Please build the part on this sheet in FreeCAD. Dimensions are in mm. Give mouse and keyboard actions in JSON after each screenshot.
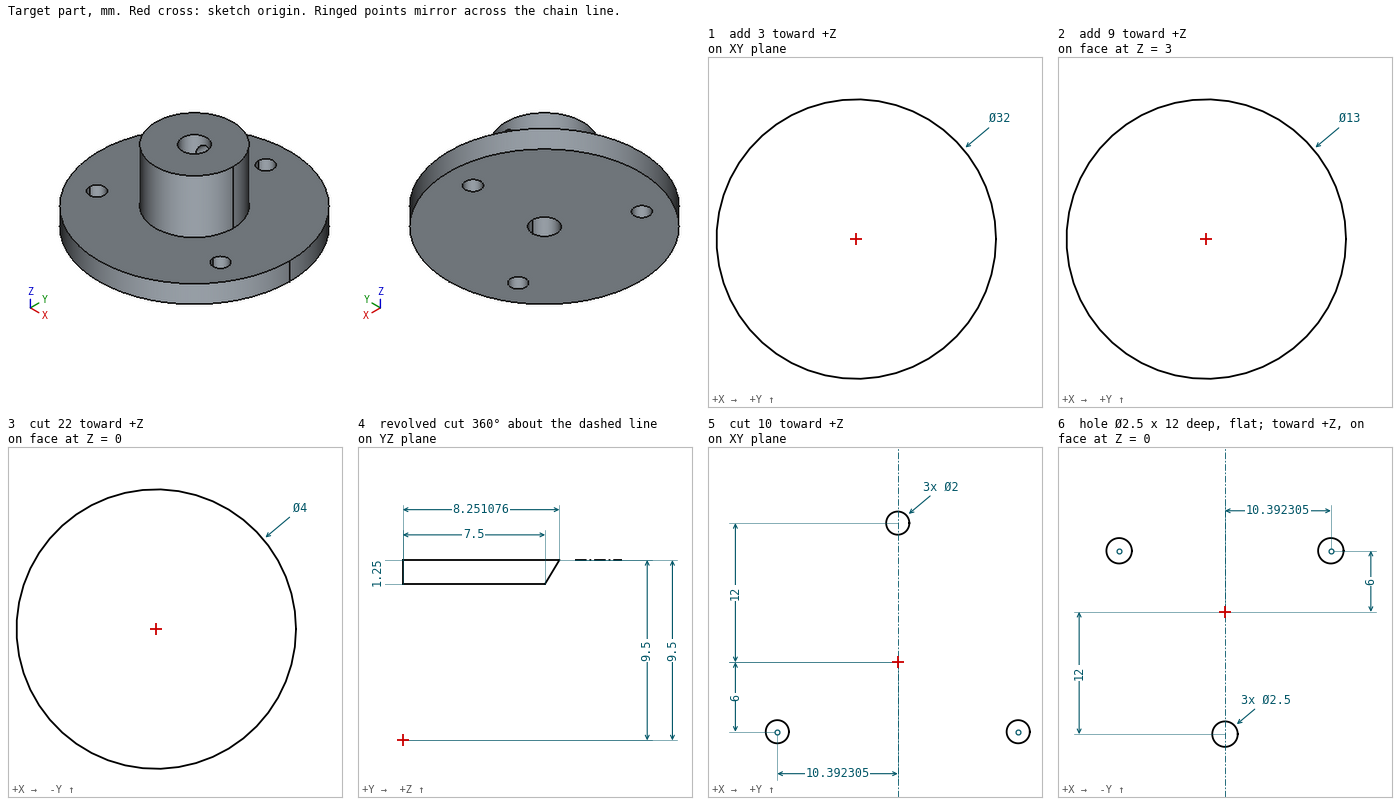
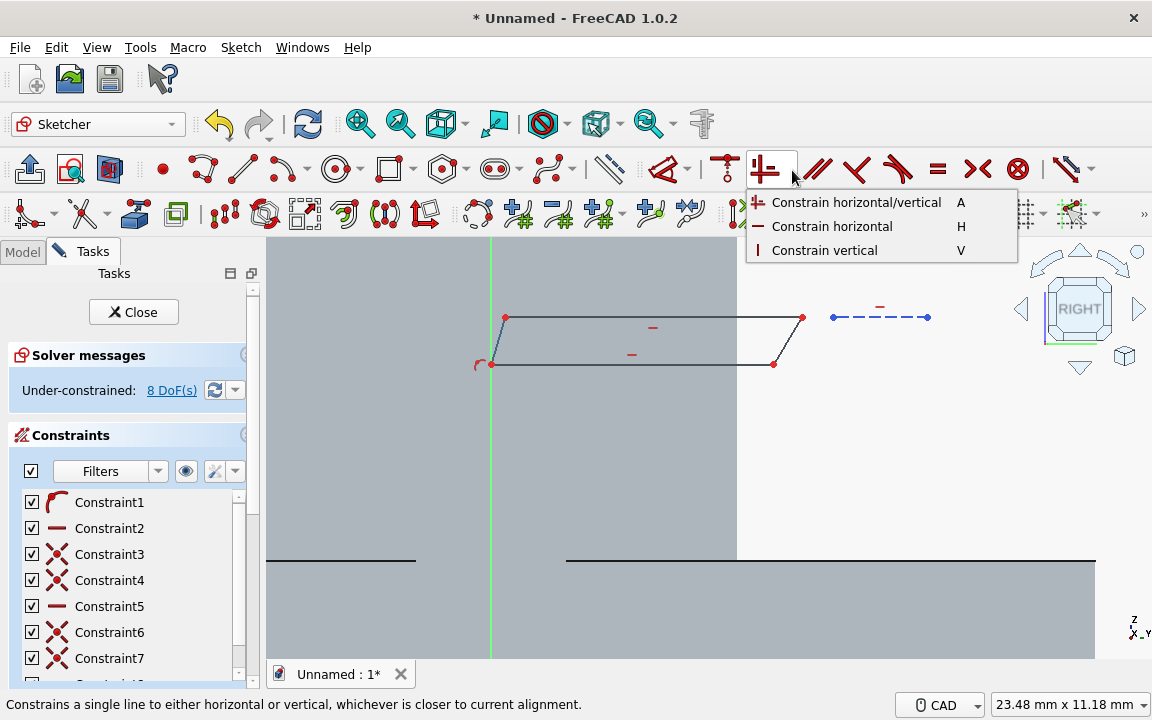
{"action": "left_click", "coordinate": [882, 250]}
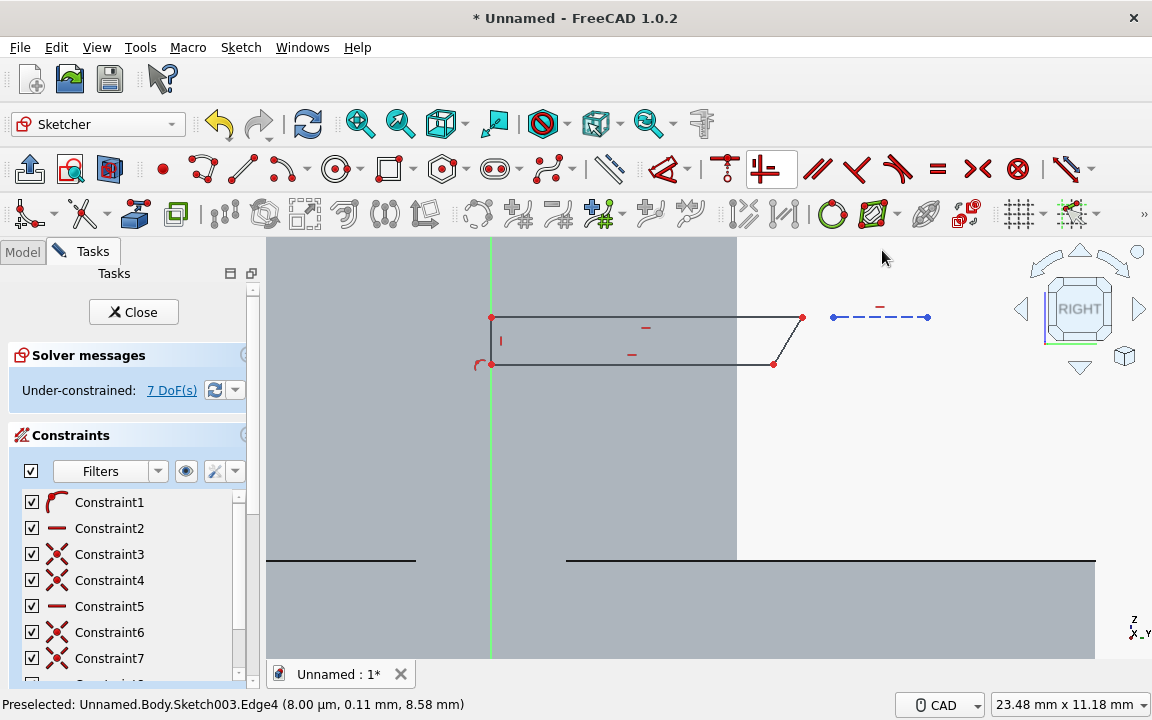
{"action": "left_click", "coordinate": [664, 170]}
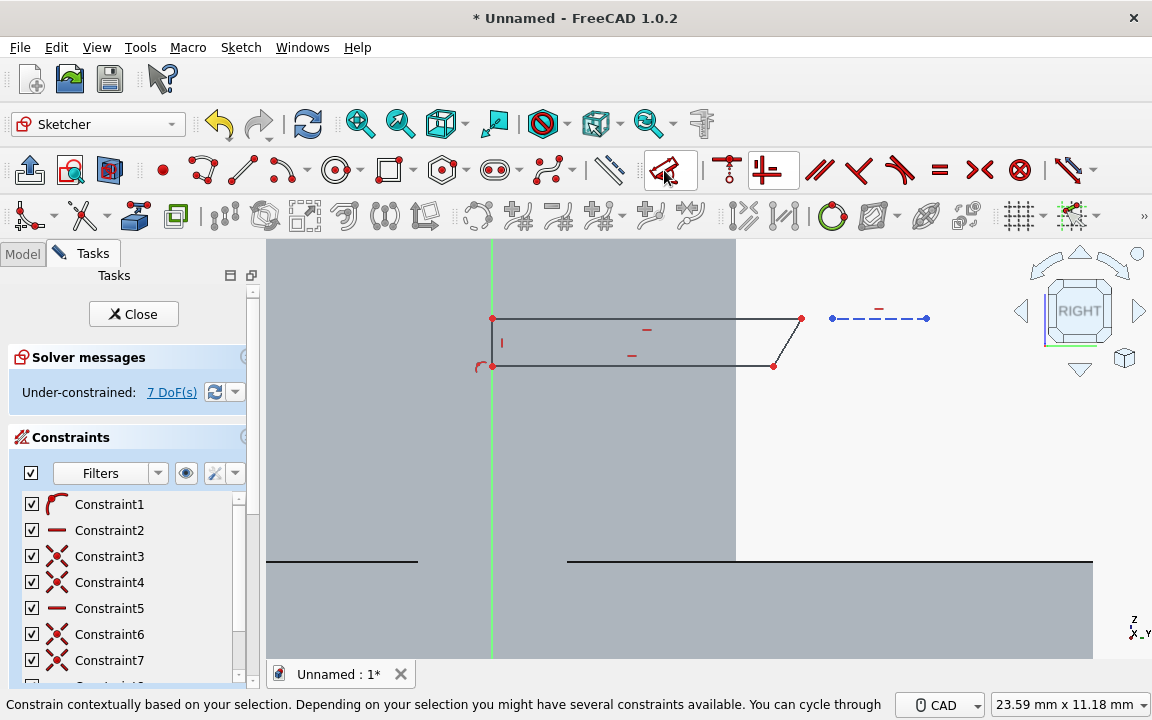
{"action": "left_click", "coordinate": [577, 366]}
{"action": "left_click", "coordinate": [633, 332]}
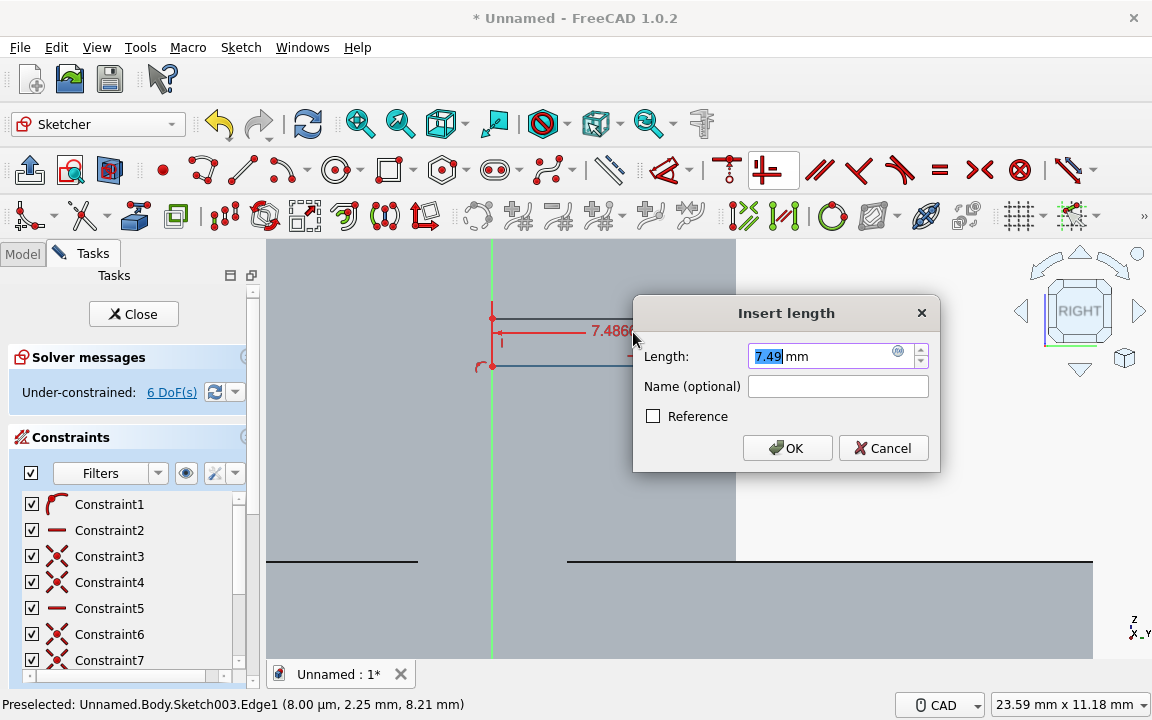
{"action": "type", "text": "7.5"}
{"action": "key", "text": "Return"}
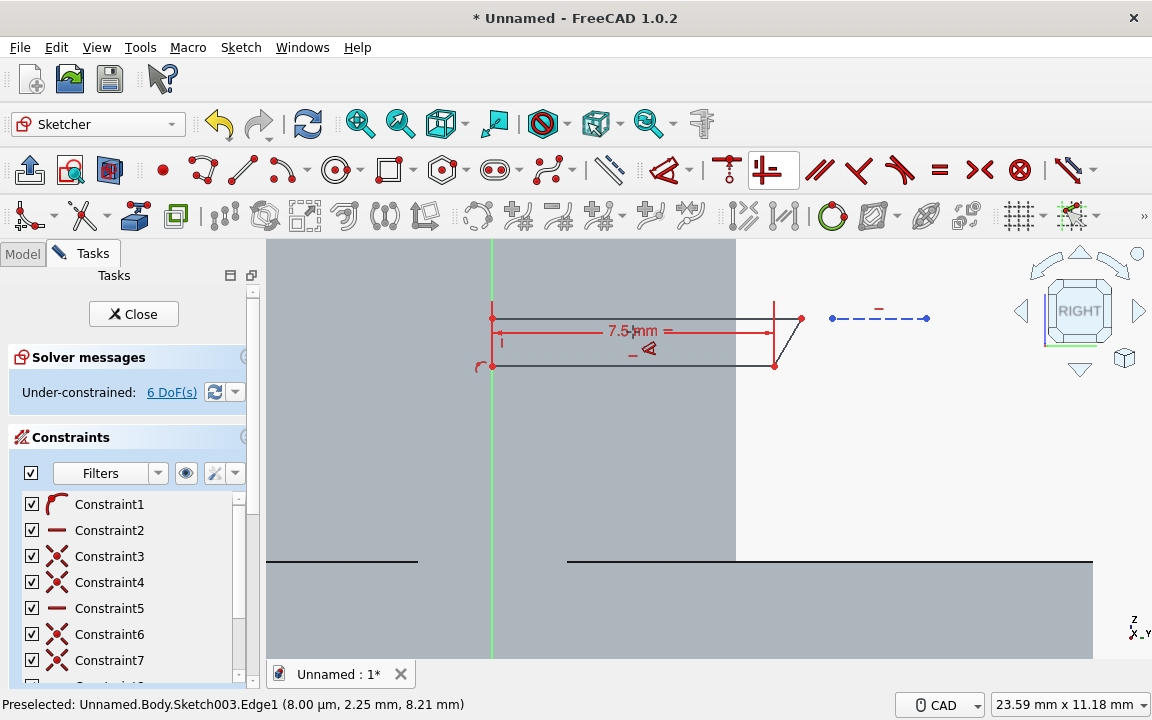
{"action": "left_click", "coordinate": [492, 333]}
{"action": "left_click", "coordinate": [458, 342]}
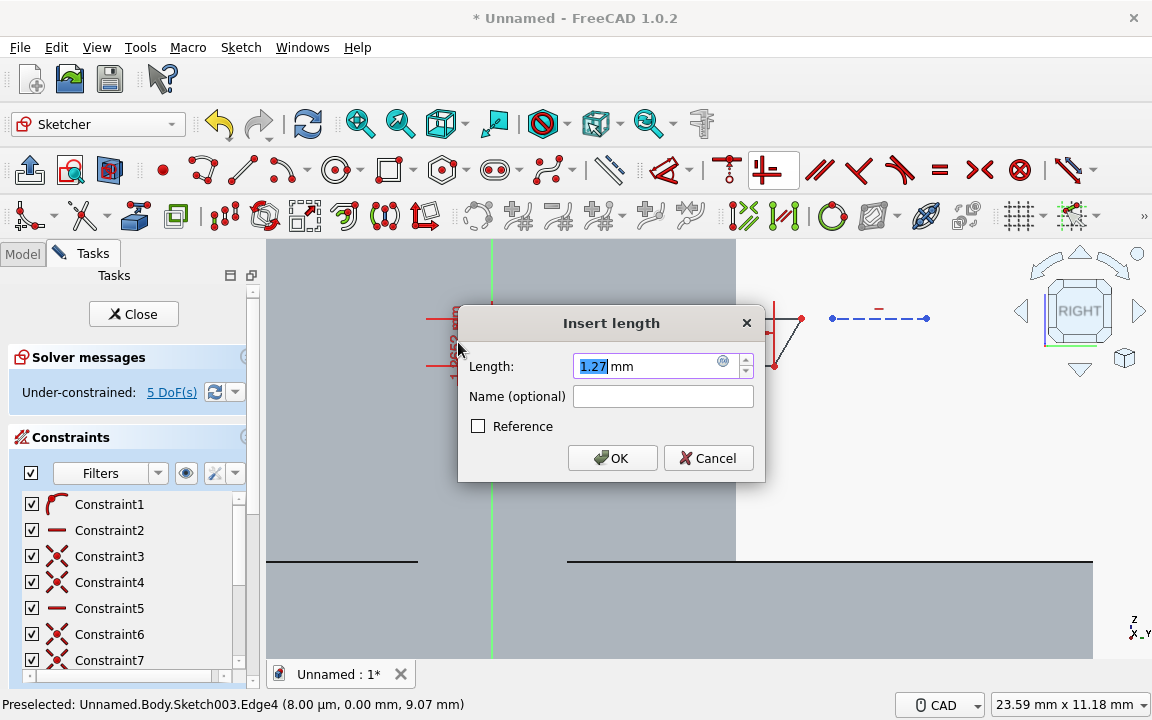
{"action": "type", "text": "1.25"}
{"action": "key", "text": "Return"}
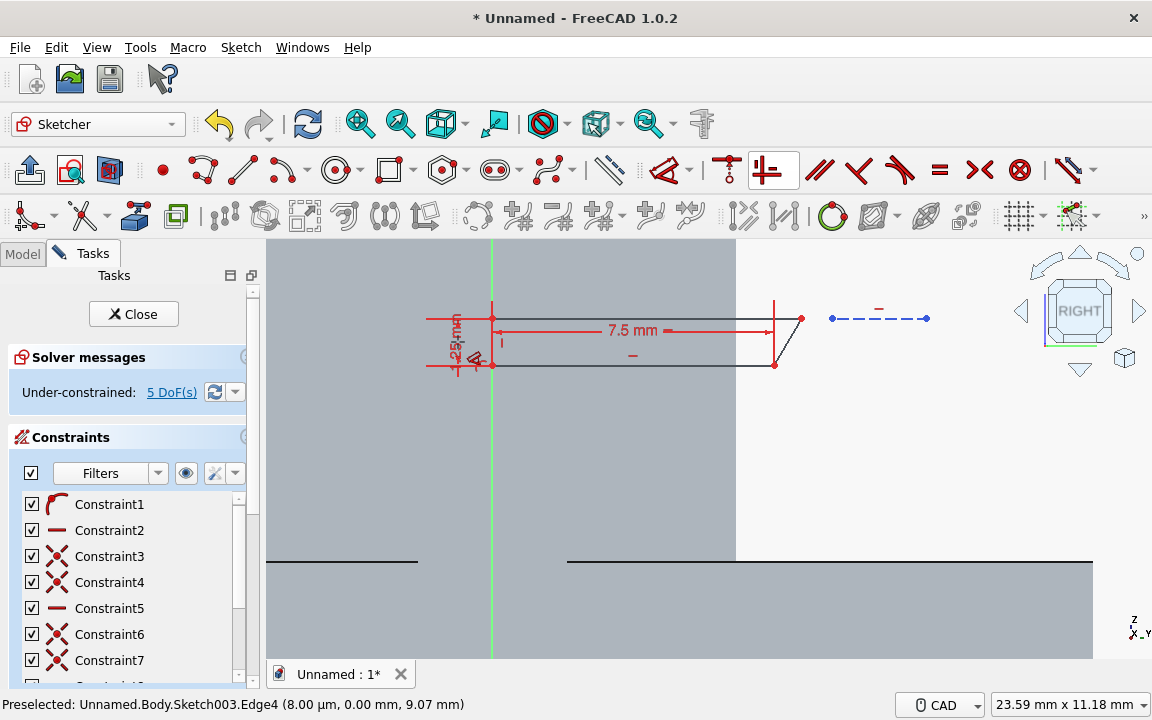
{"action": "left_click", "coordinate": [802, 319]}
{"action": "left_click", "coordinate": [458, 475]}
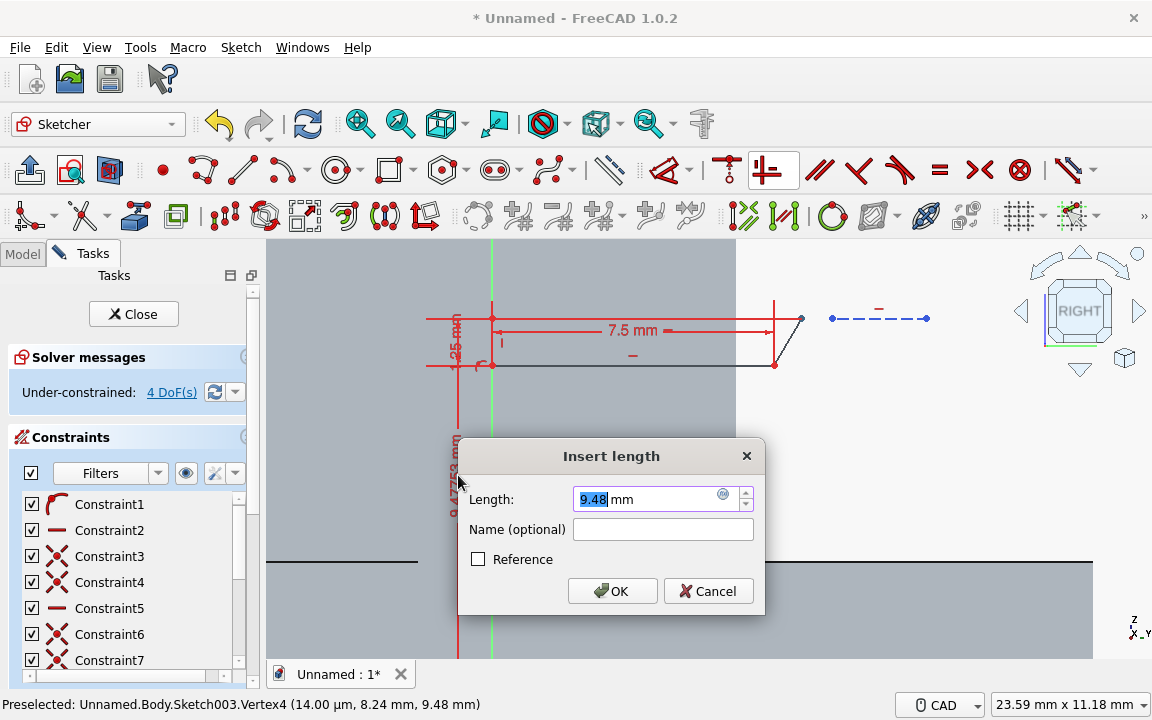
{"action": "type", "text": "9.5"}
{"action": "key", "text": "Return"}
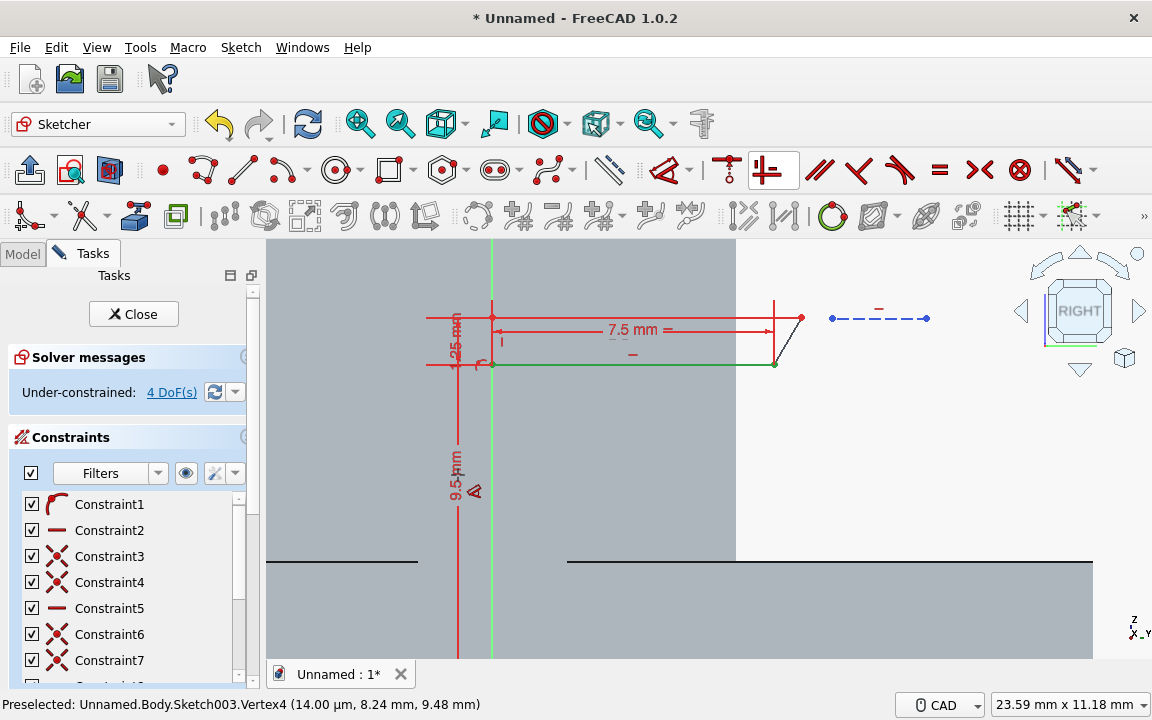
{"action": "left_click", "coordinate": [833, 319]}
{"action": "left_click", "coordinate": [458, 403]}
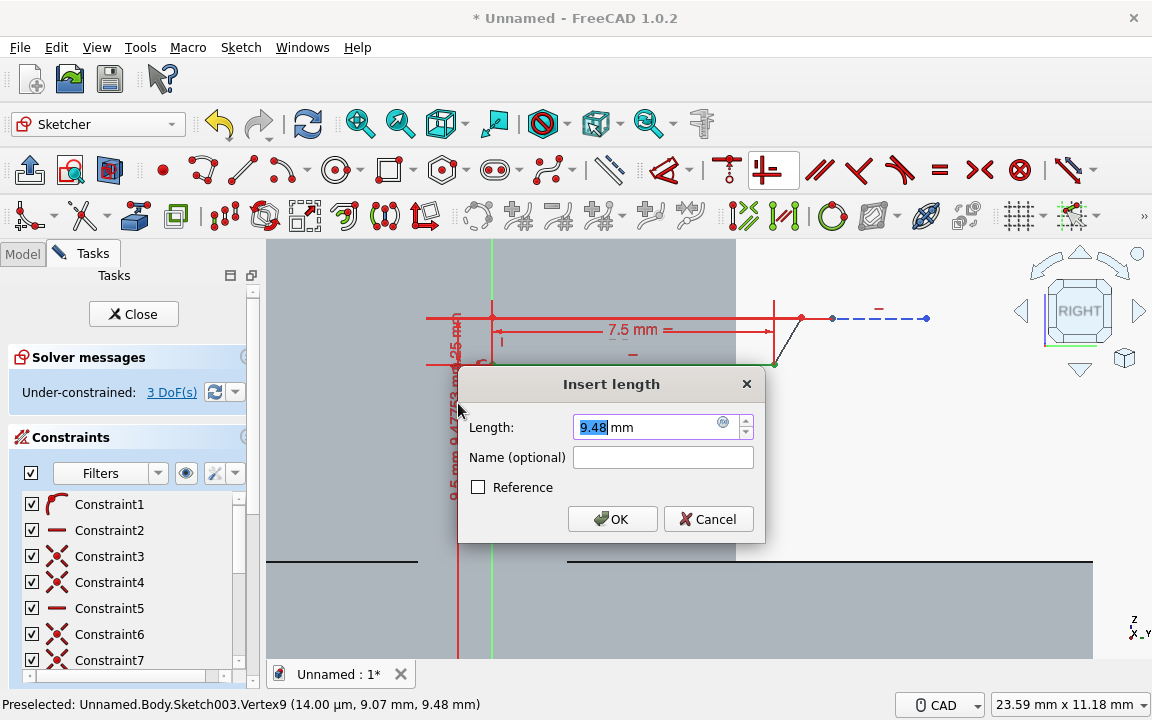
{"action": "type", "text": "9.5"}
{"action": "key", "text": "Return"}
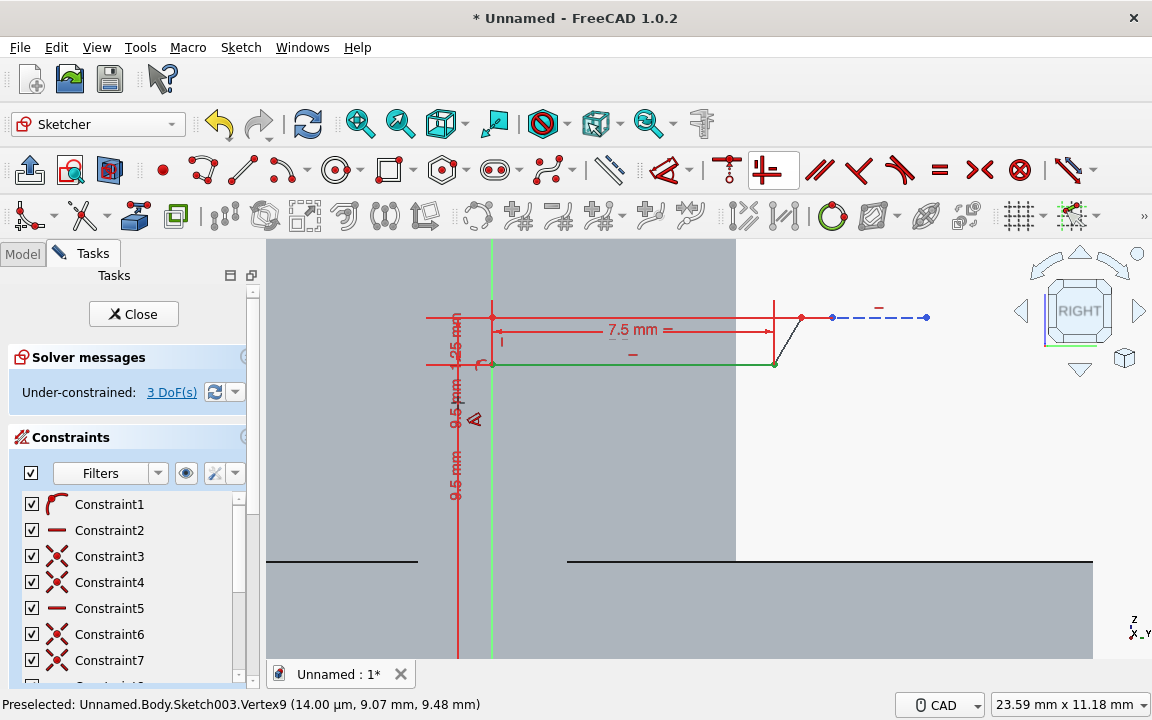
{"action": "left_click", "coordinate": [709, 318]}
{"action": "left_click", "coordinate": [647, 284]}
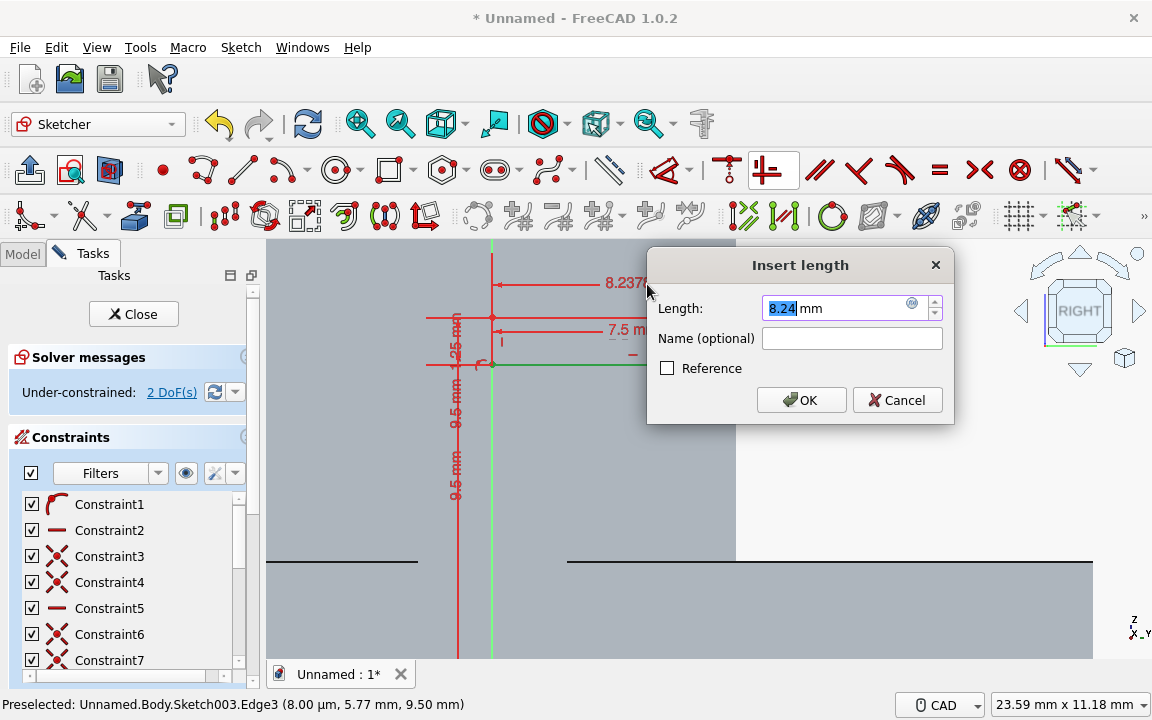
{"action": "type", "text": "8.251076"}
{"action": "key", "text": "Return"}
{"action": "key", "text": "Escape"}